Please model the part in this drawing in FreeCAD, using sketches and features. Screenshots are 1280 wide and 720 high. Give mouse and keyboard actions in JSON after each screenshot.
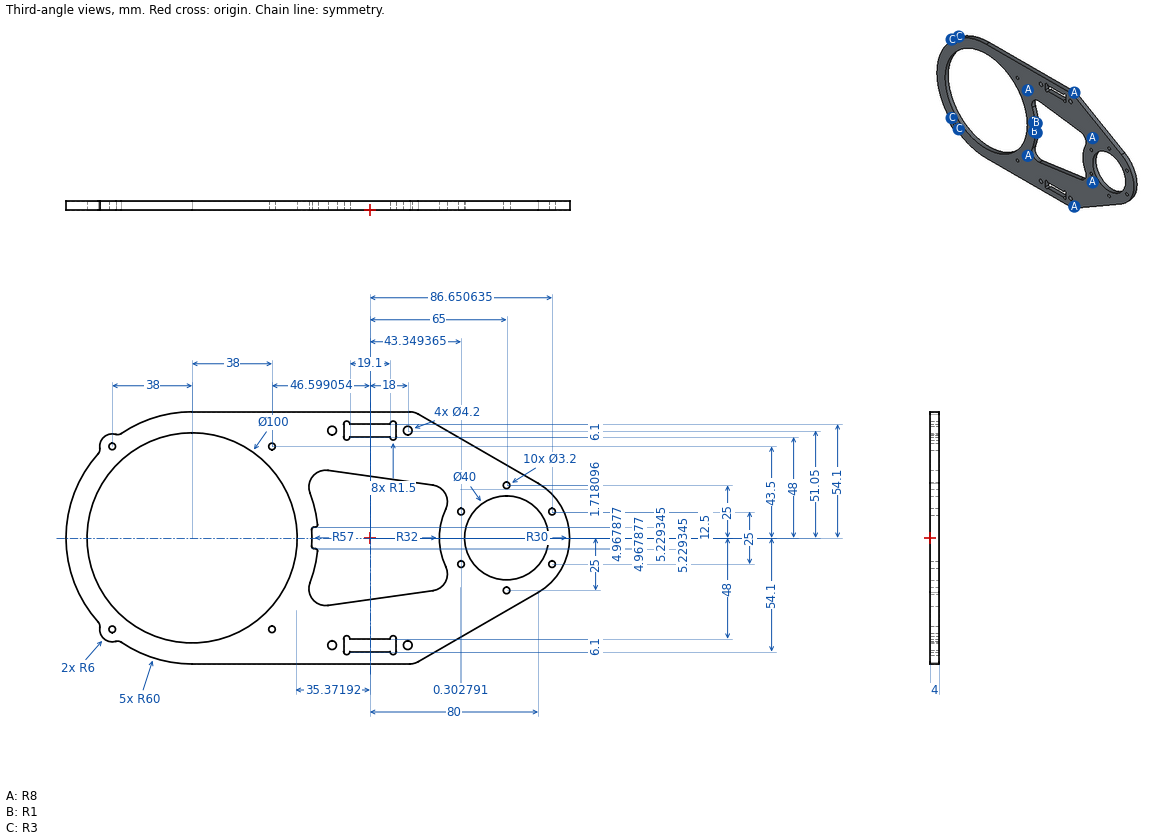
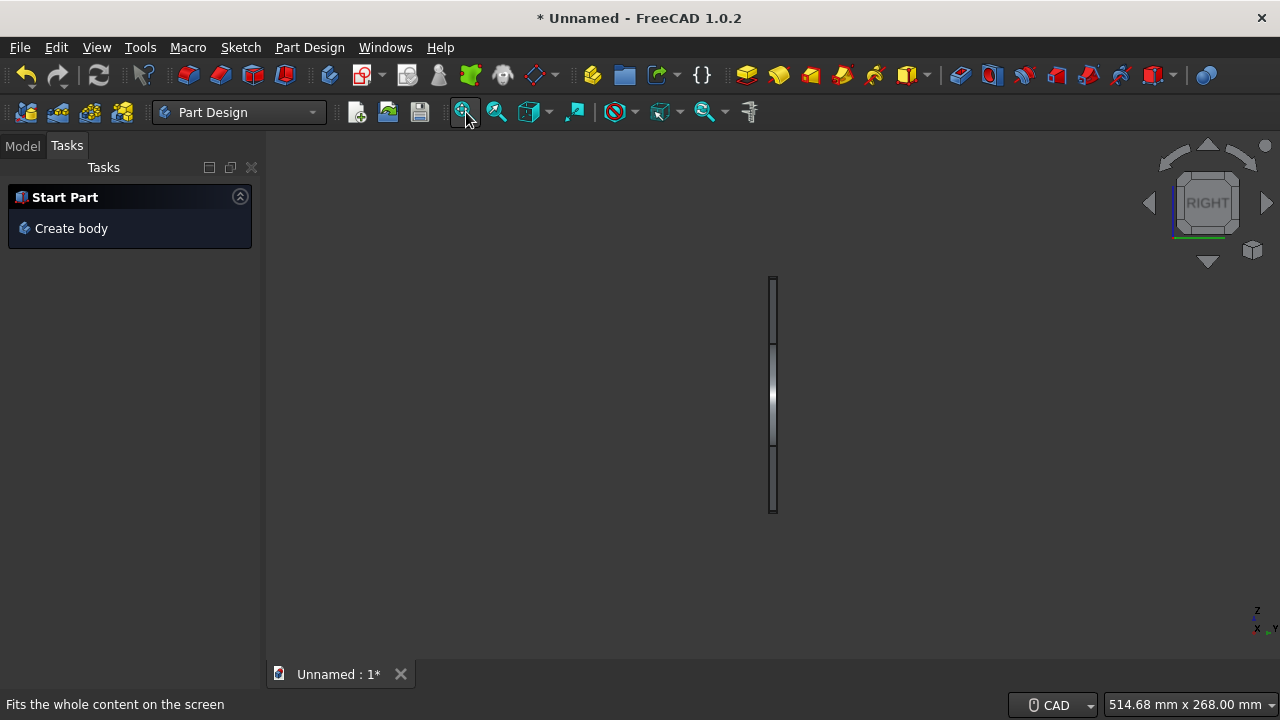
{"action": "left_click", "coordinate": [466, 112]}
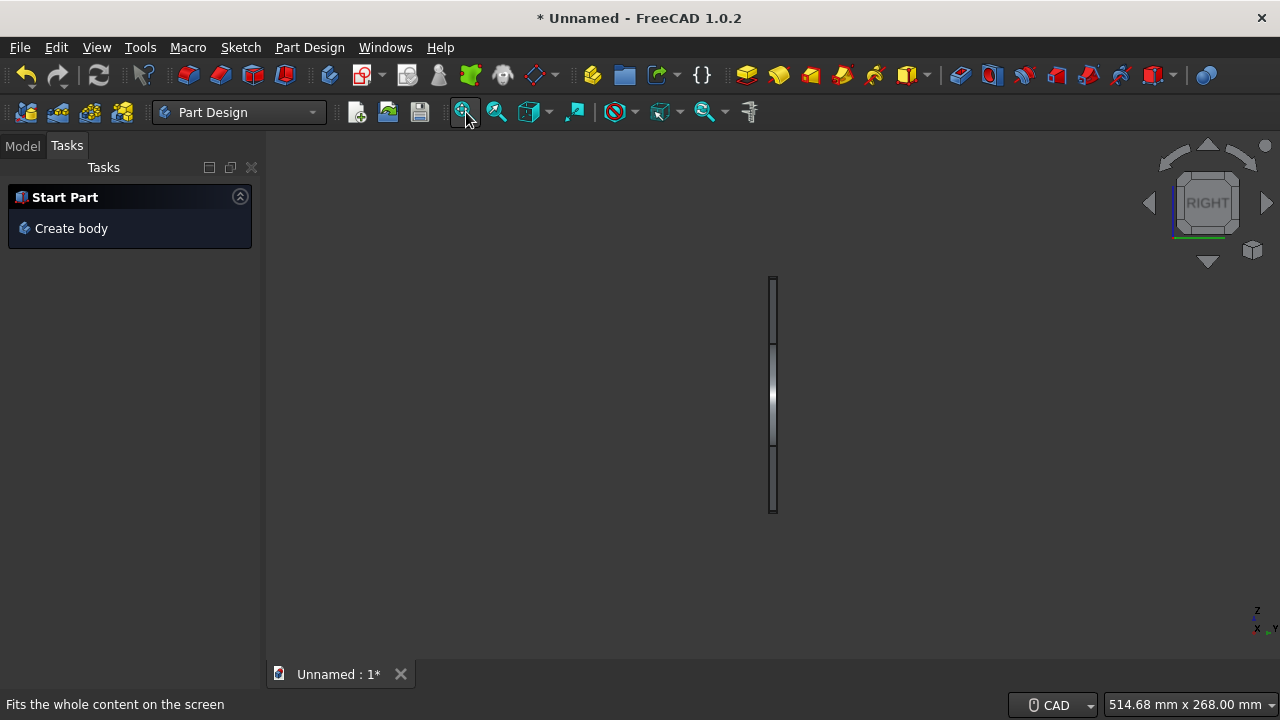
{"action": "scroll", "coordinate": [773, 298], "scroll_direction": "up", "scroll_amount": 9}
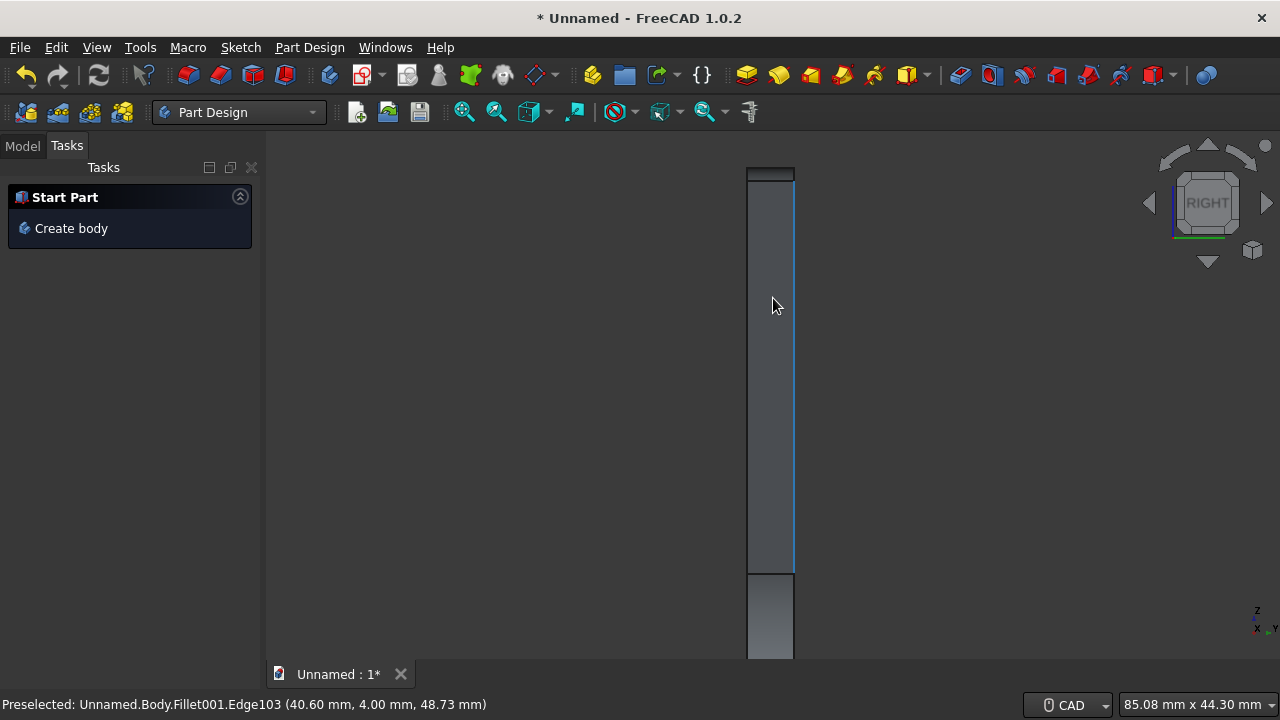
{"action": "left_click", "coordinate": [466, 112]}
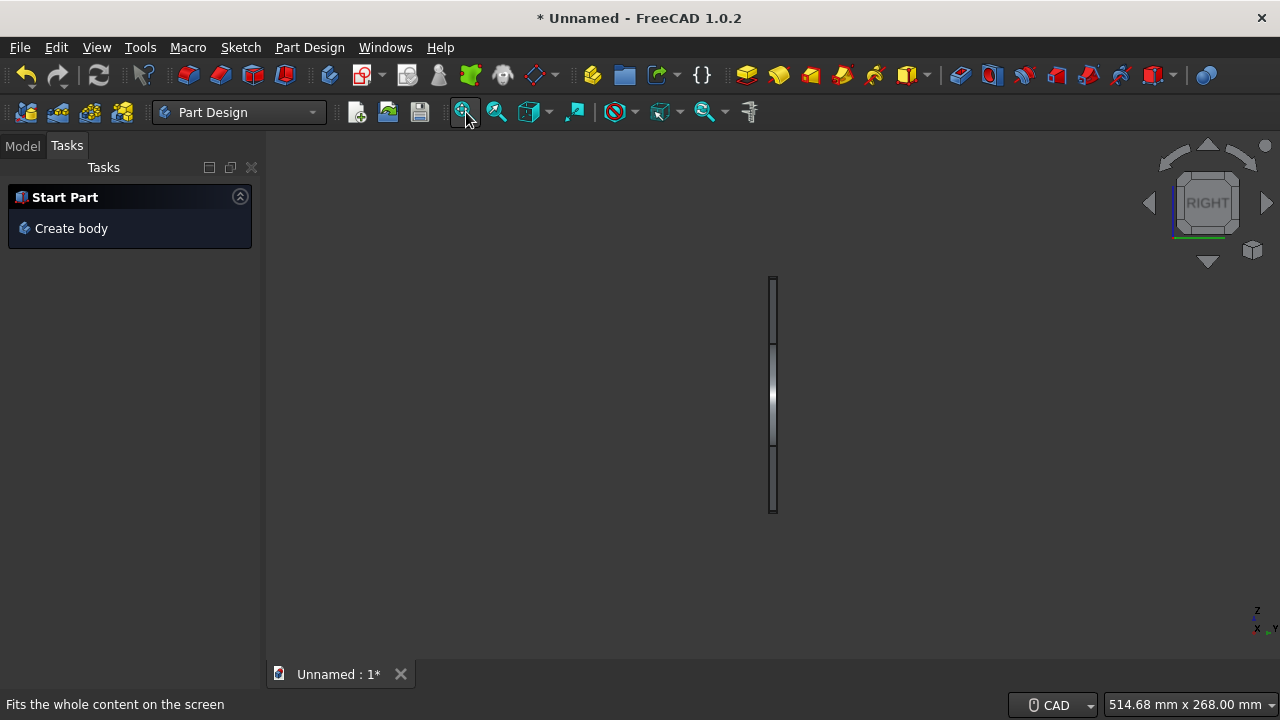
{"action": "key", "text": "5"}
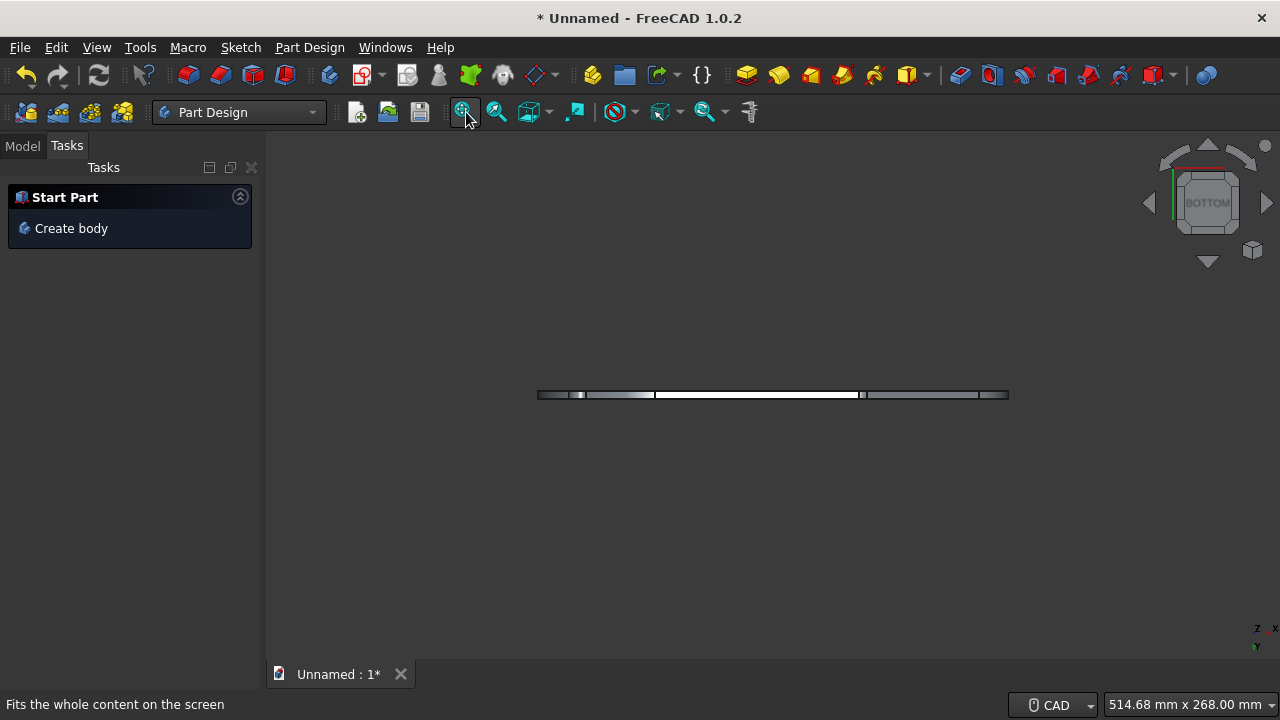
{"action": "scroll", "coordinate": [586, 394], "scroll_direction": "up", "scroll_amount": 9}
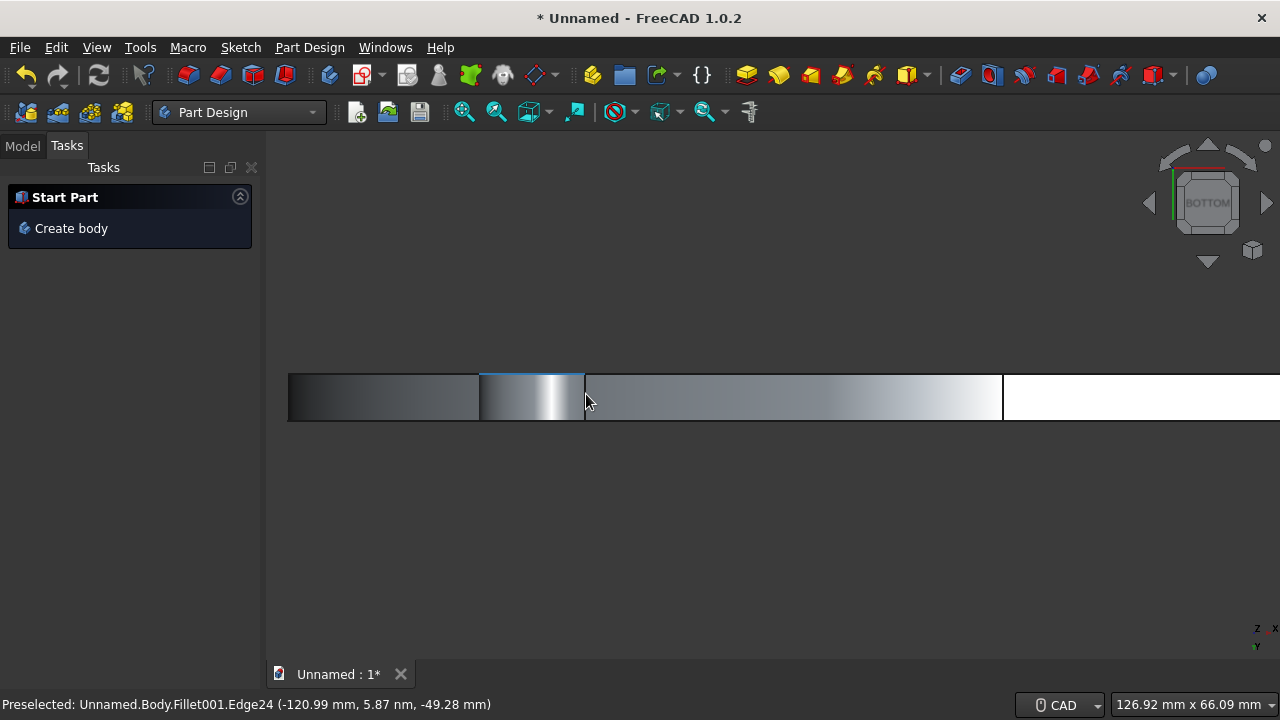
{"action": "left_click", "coordinate": [466, 112]}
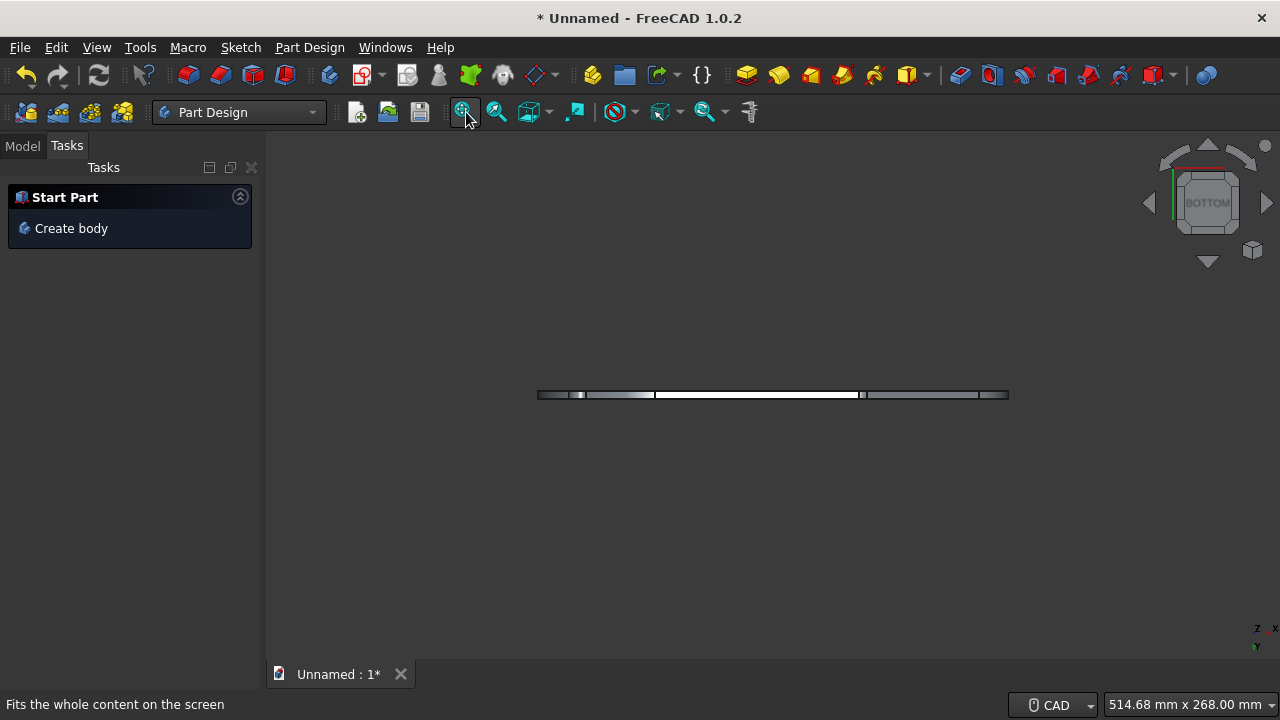
{"action": "key", "text": "4"}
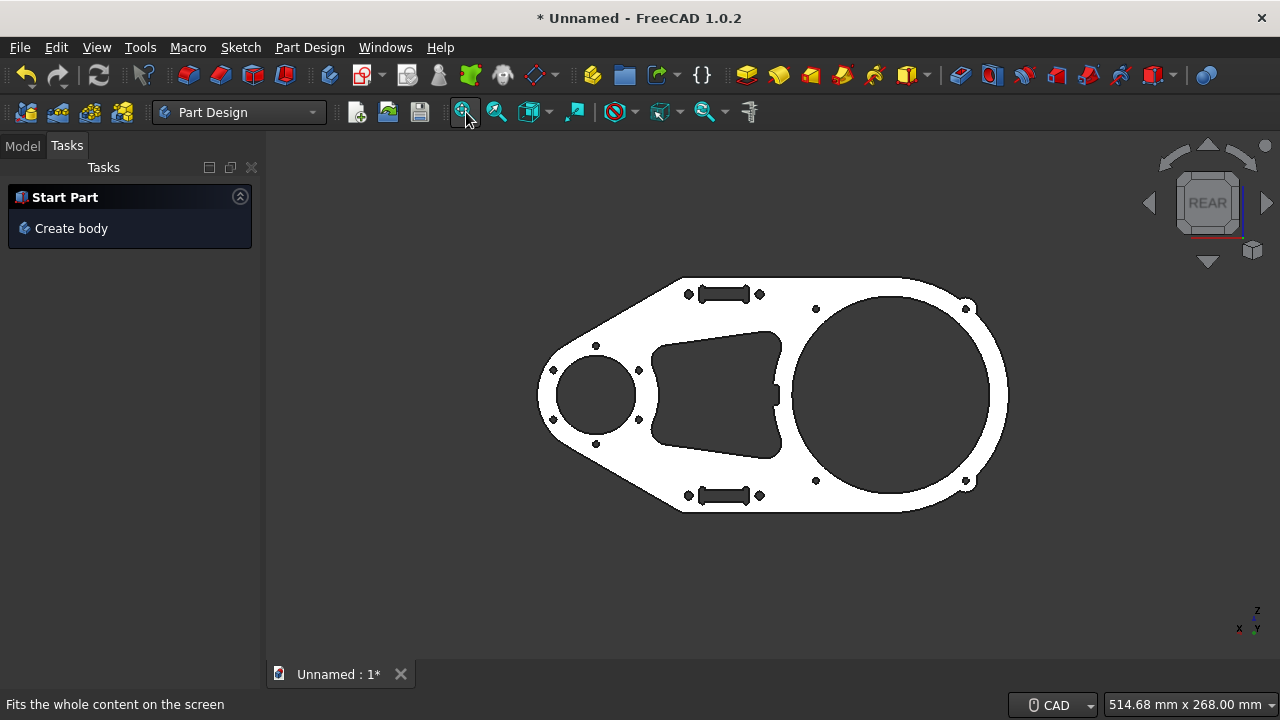
{"action": "scroll", "coordinate": [960, 298], "scroll_direction": "up", "scroll_amount": 9}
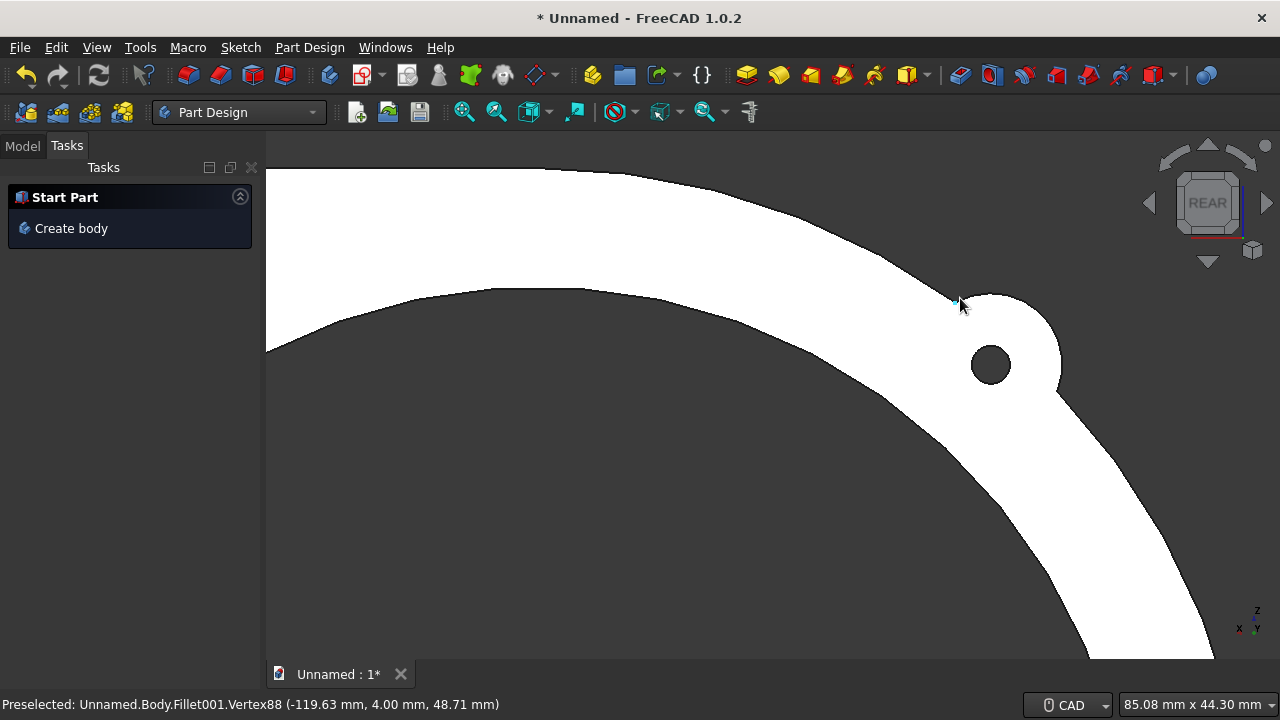
{"action": "key", "text": "v f"}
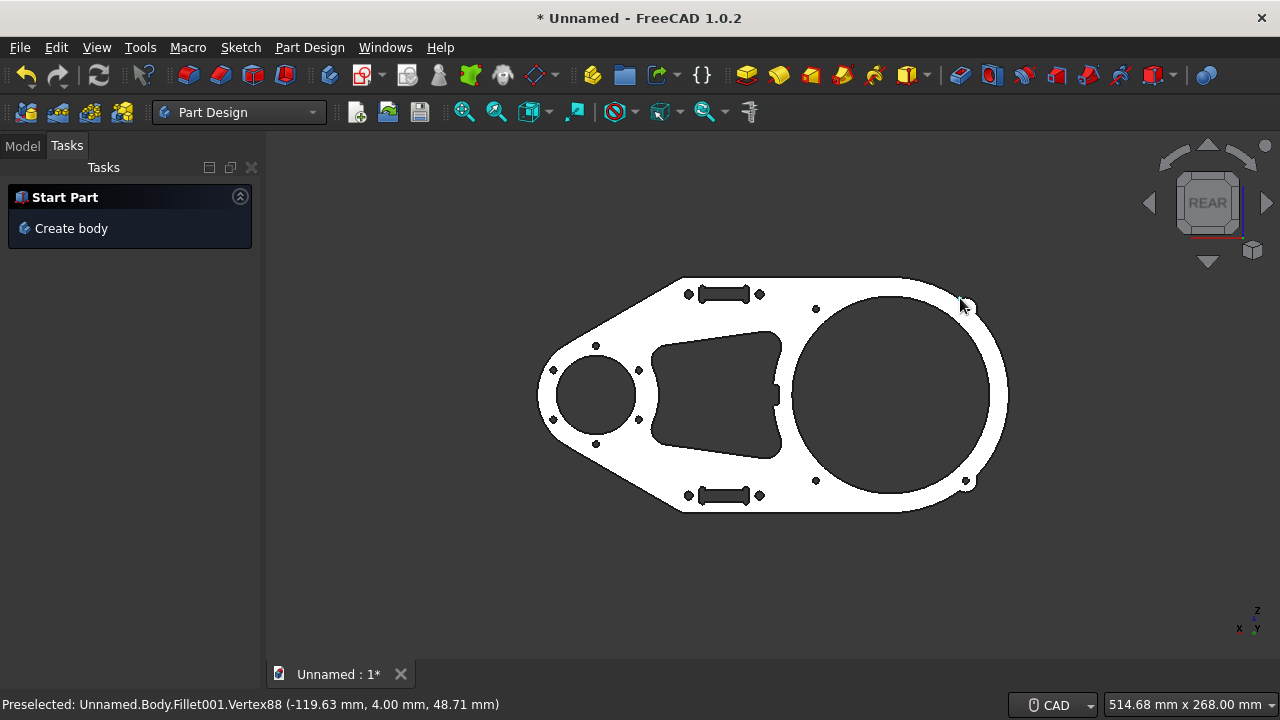
{"action": "key", "text": "6"}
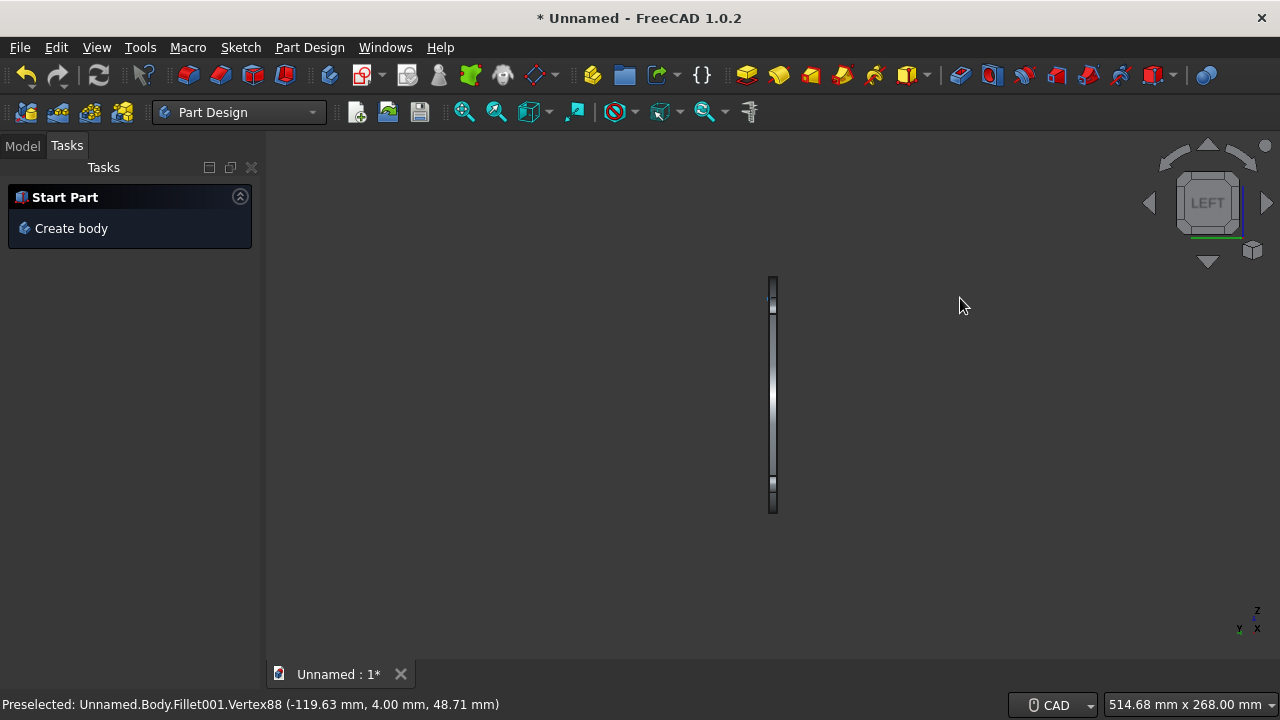
{"action": "left_click", "coordinate": [466, 112]}